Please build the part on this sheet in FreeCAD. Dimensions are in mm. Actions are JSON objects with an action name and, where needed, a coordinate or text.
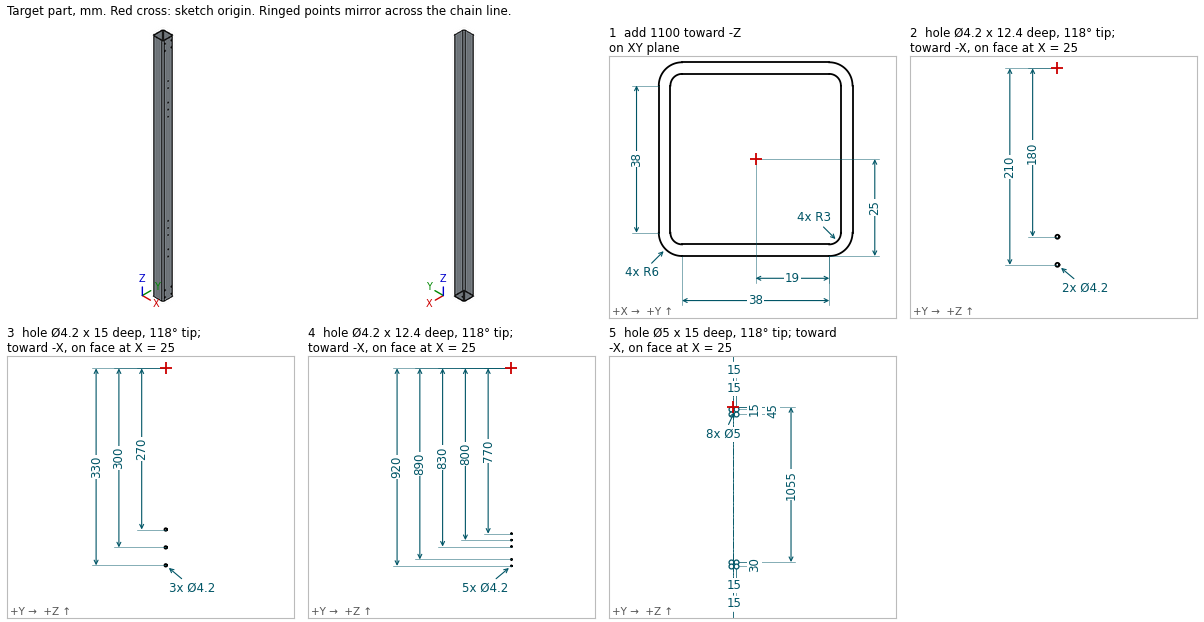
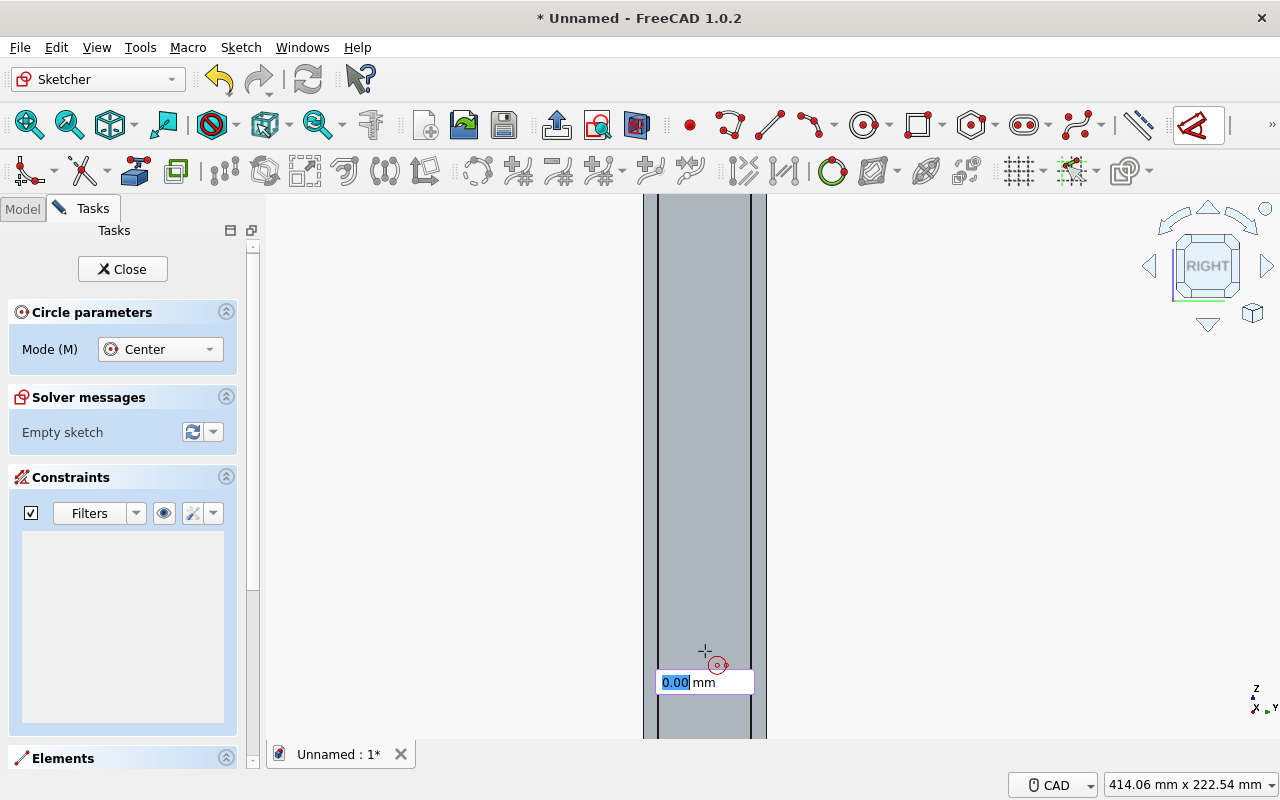
{"action": "scroll", "coordinate": [710, 649], "scroll_direction": "up", "scroll_amount": 6}
{"action": "mouse_move", "coordinate": [708, 646]}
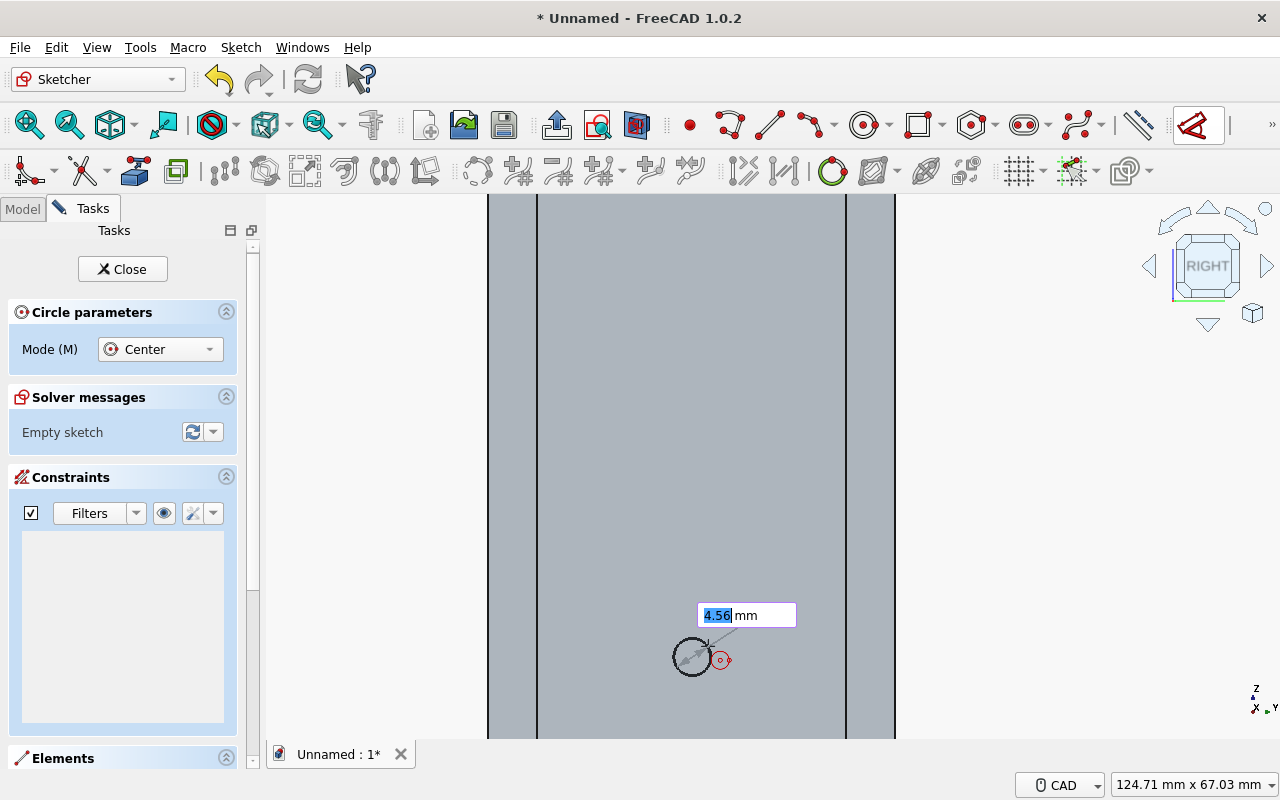
{"action": "type", "text": "4.2"}
{"action": "key", "text": "Return"}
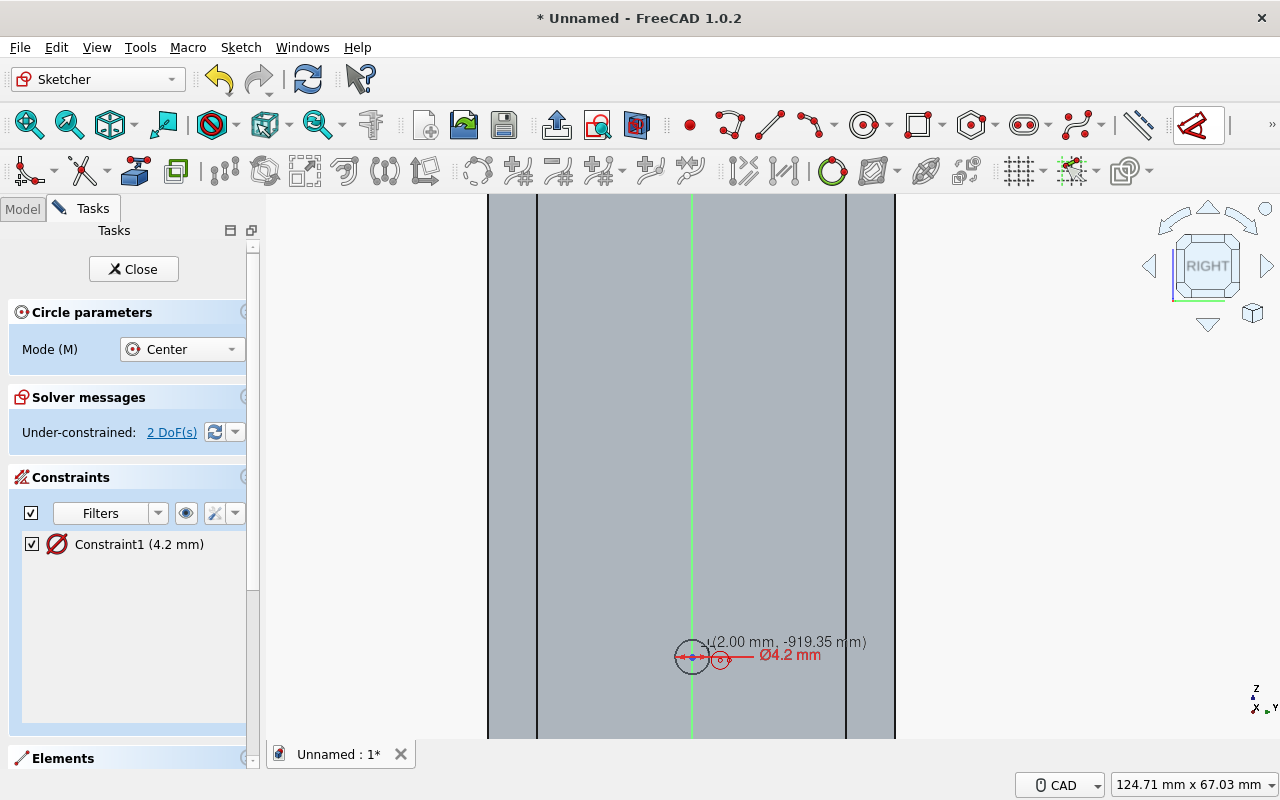
{"action": "scroll", "coordinate": [692, 408], "scroll_direction": "up", "scroll_amount": 2}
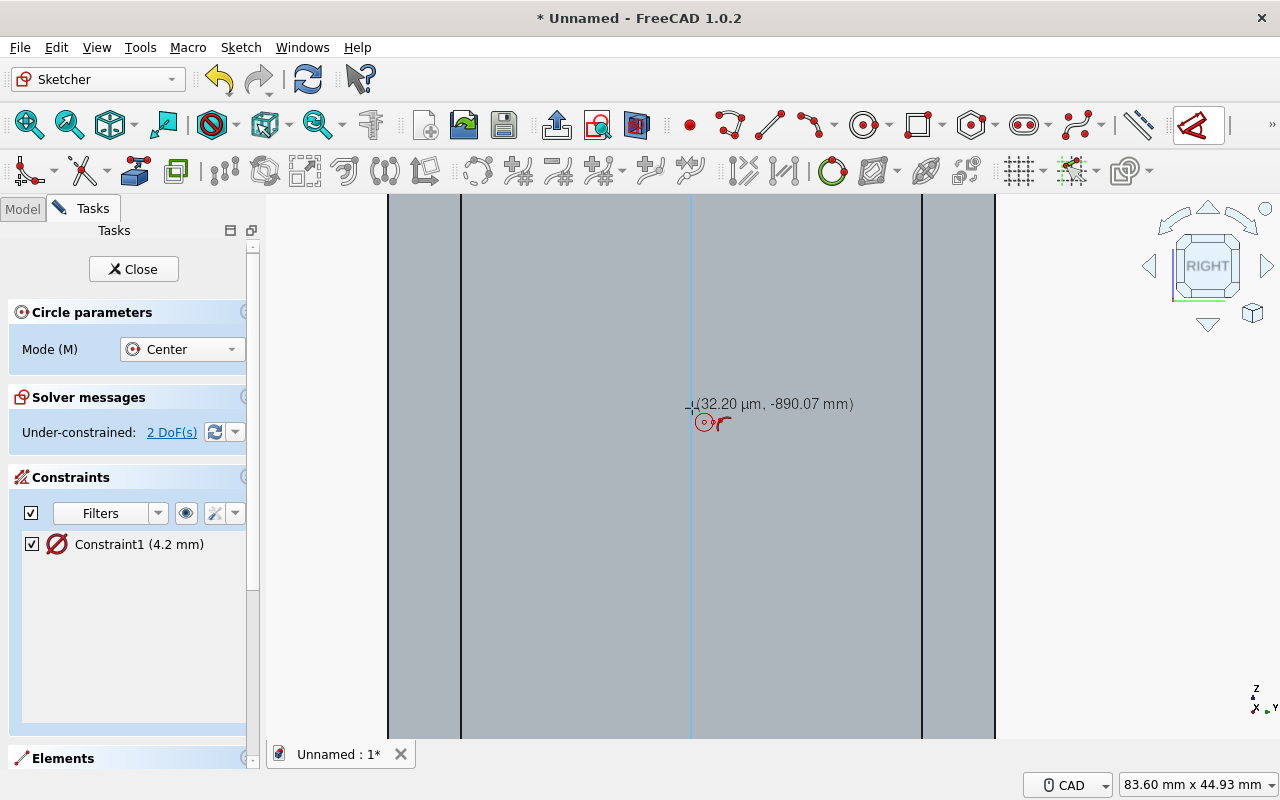
{"action": "scroll", "coordinate": [708, 619], "scroll_direction": "down", "scroll_amount": 8}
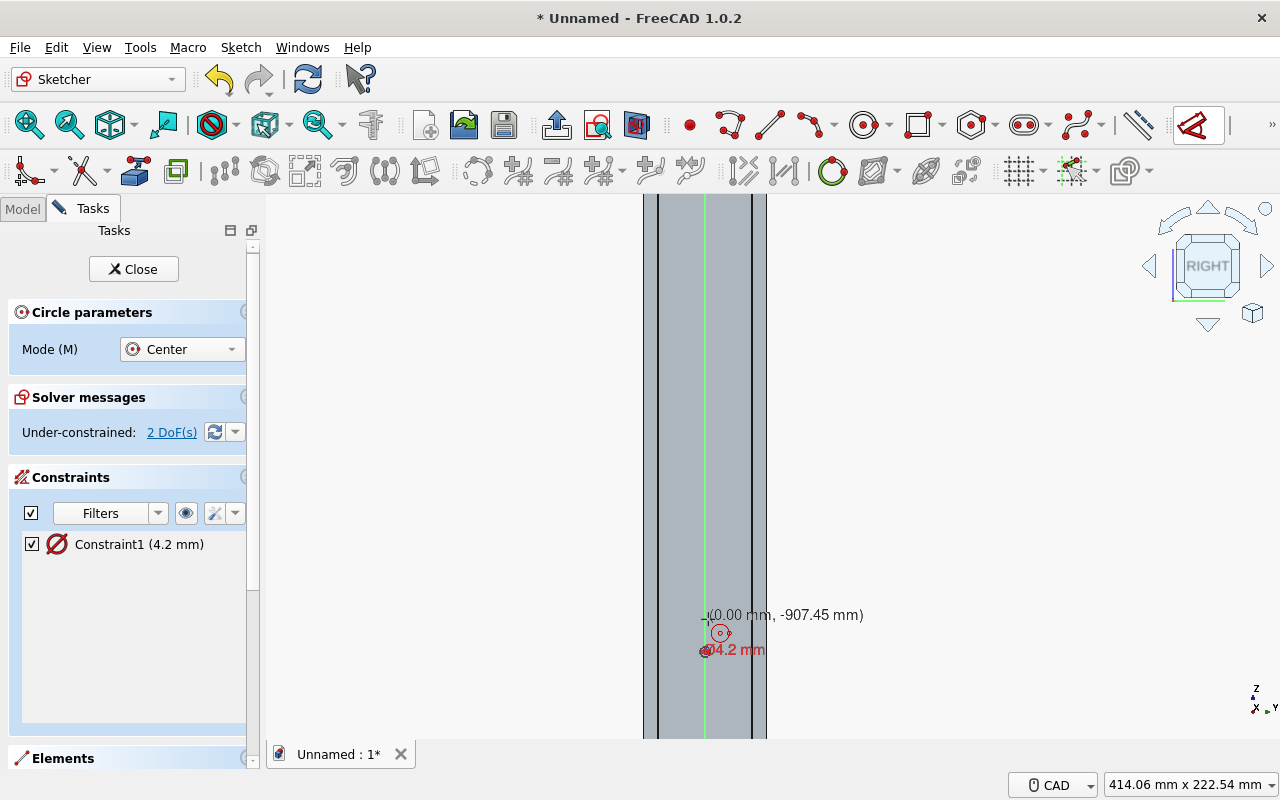
{"action": "left_click", "coordinate": [705, 577]}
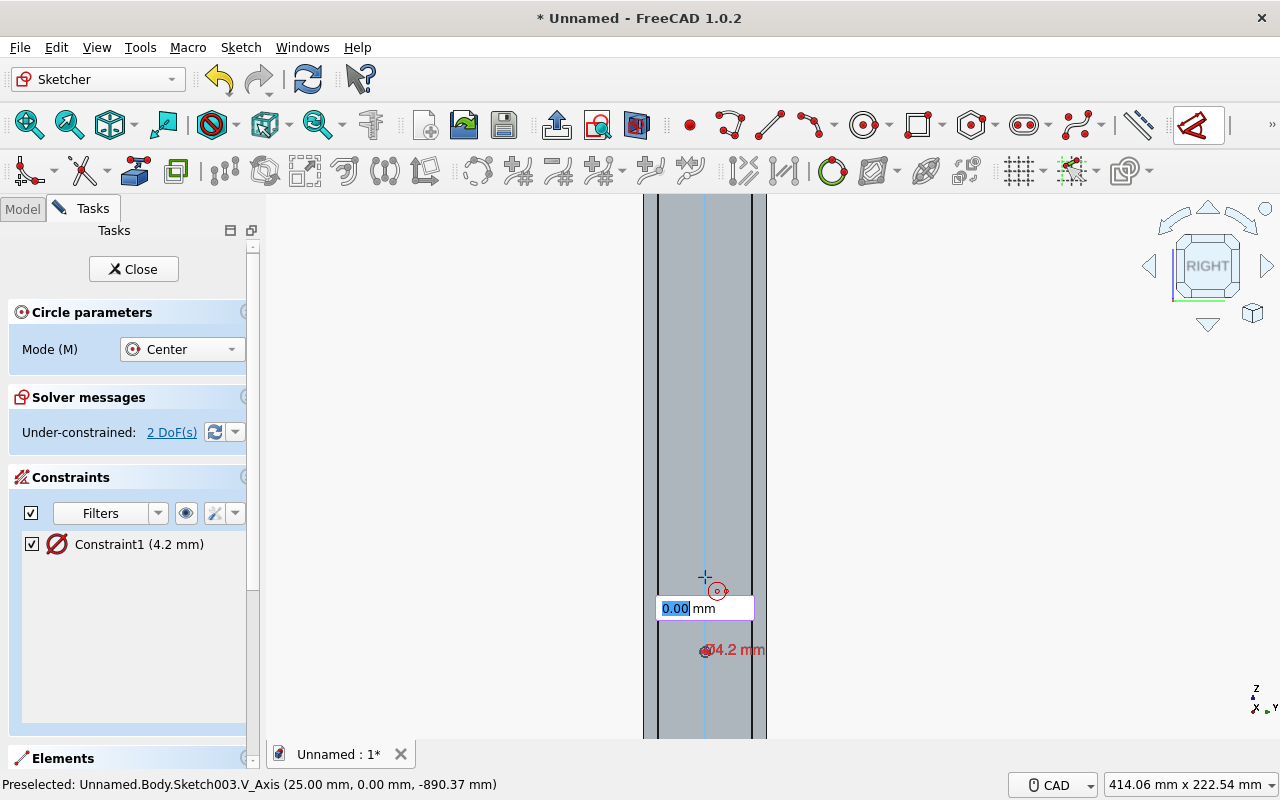
{"action": "scroll", "coordinate": [710, 575], "scroll_direction": "up", "scroll_amount": 6}
{"action": "mouse_move", "coordinate": [708, 575]}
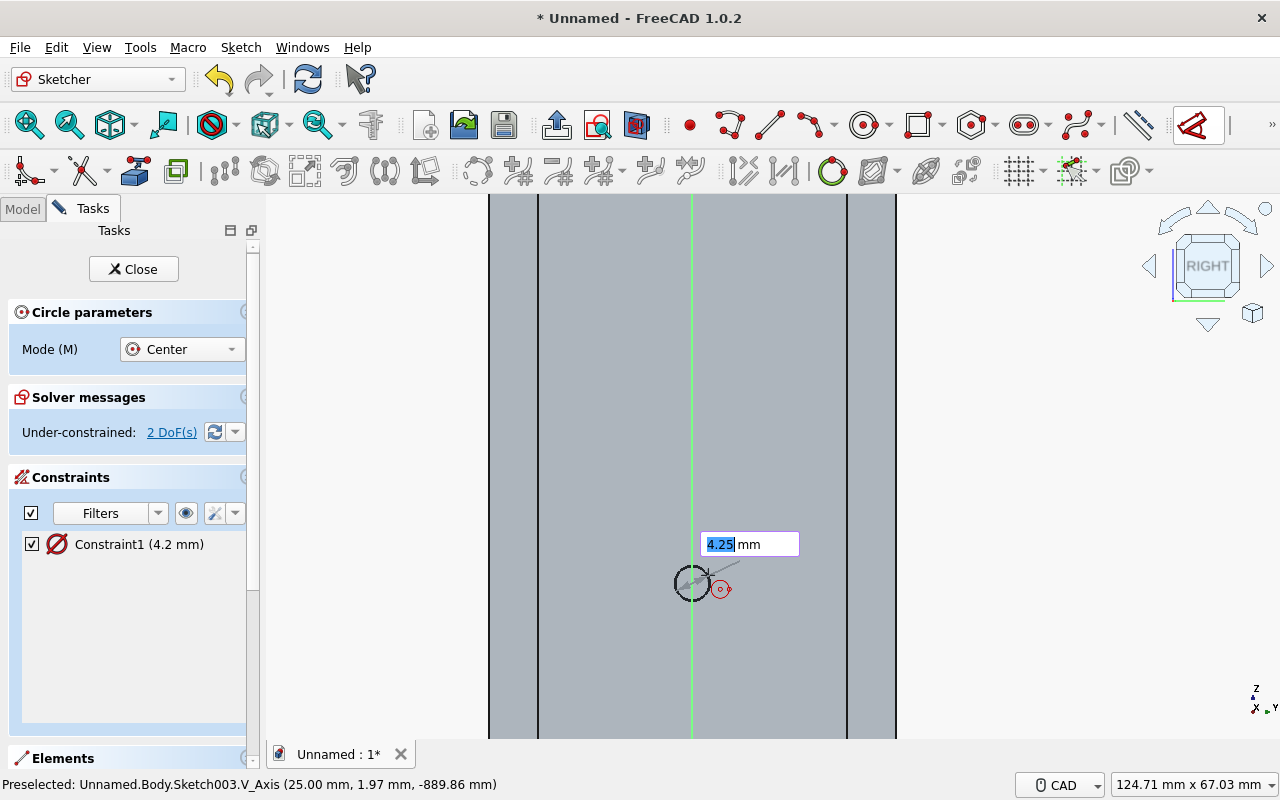
{"action": "type", "text": "4.2"}
{"action": "key", "text": "Return"}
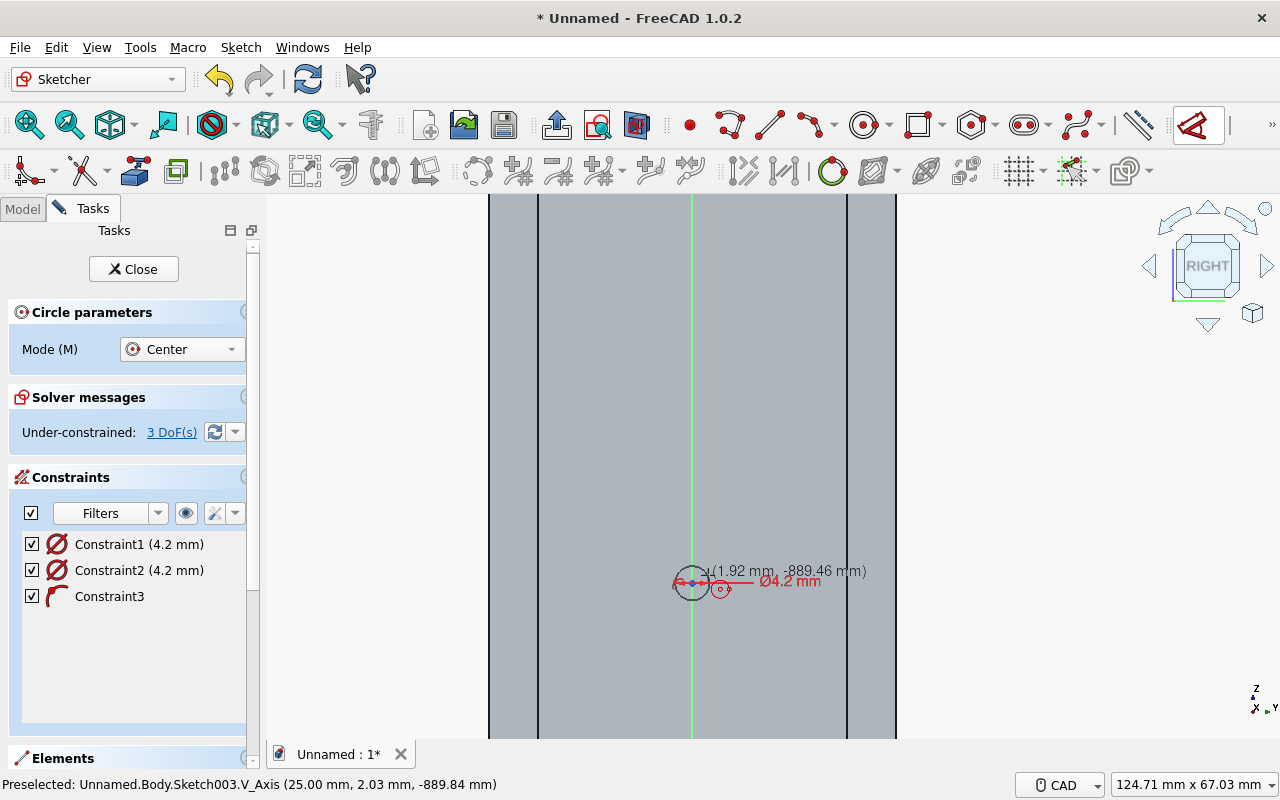
{"action": "scroll", "coordinate": [710, 575], "scroll_direction": "down", "scroll_amount": 6}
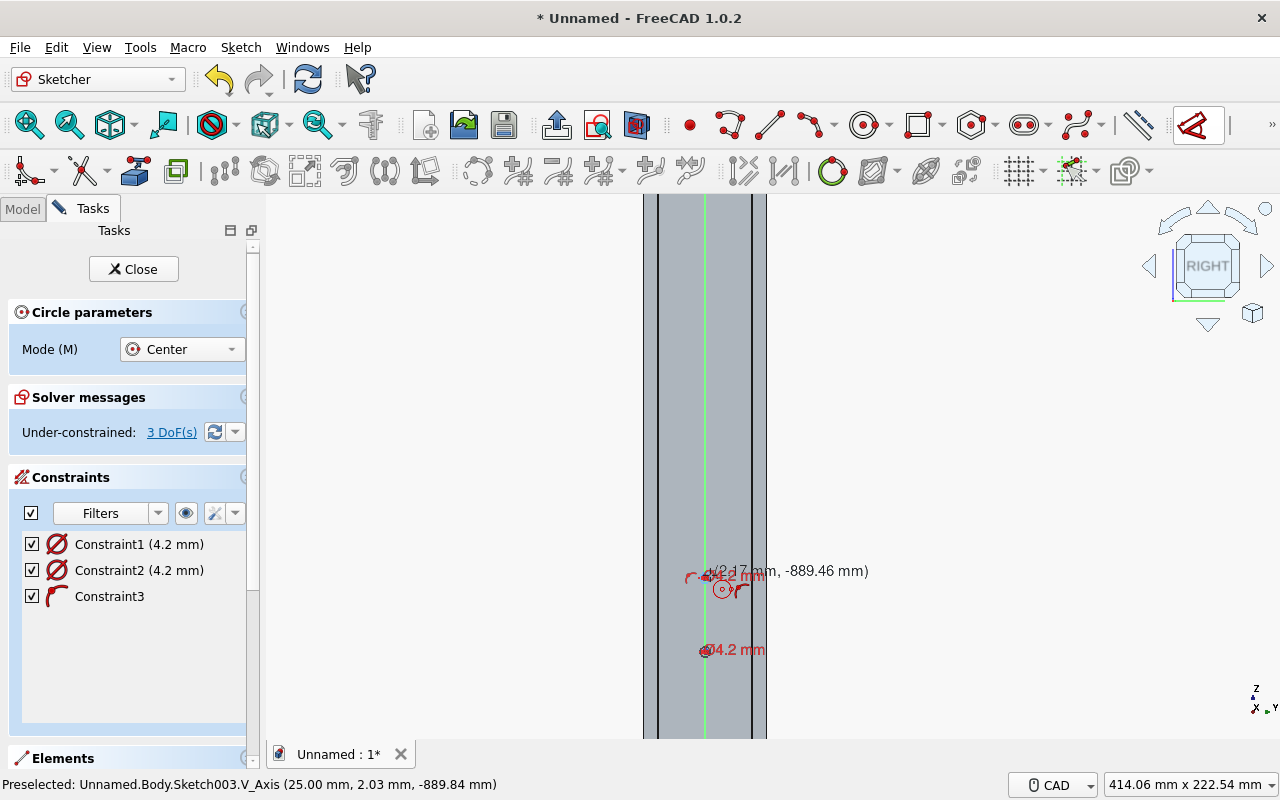
{"action": "scroll", "coordinate": [705, 430], "scroll_direction": "up", "scroll_amount": 8}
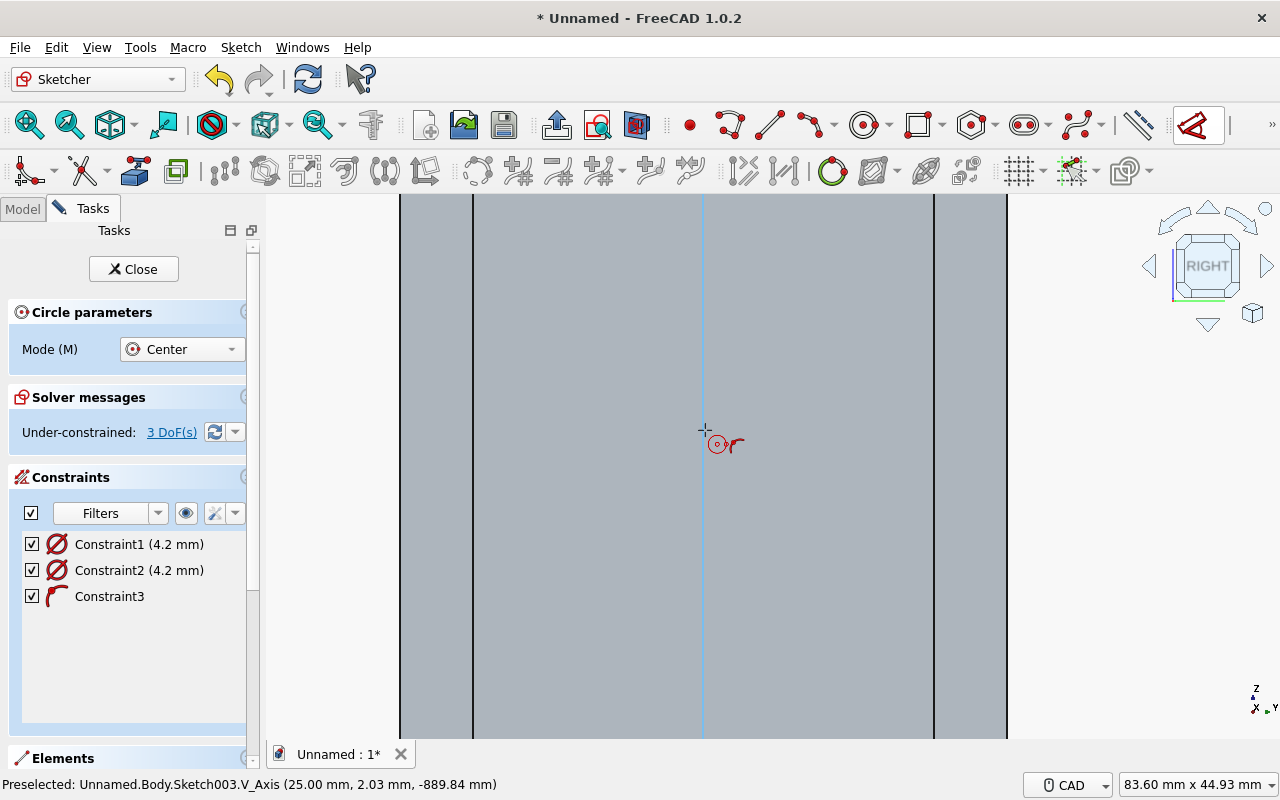
{"action": "scroll", "coordinate": [705, 430], "scroll_direction": "down", "scroll_amount": 8}